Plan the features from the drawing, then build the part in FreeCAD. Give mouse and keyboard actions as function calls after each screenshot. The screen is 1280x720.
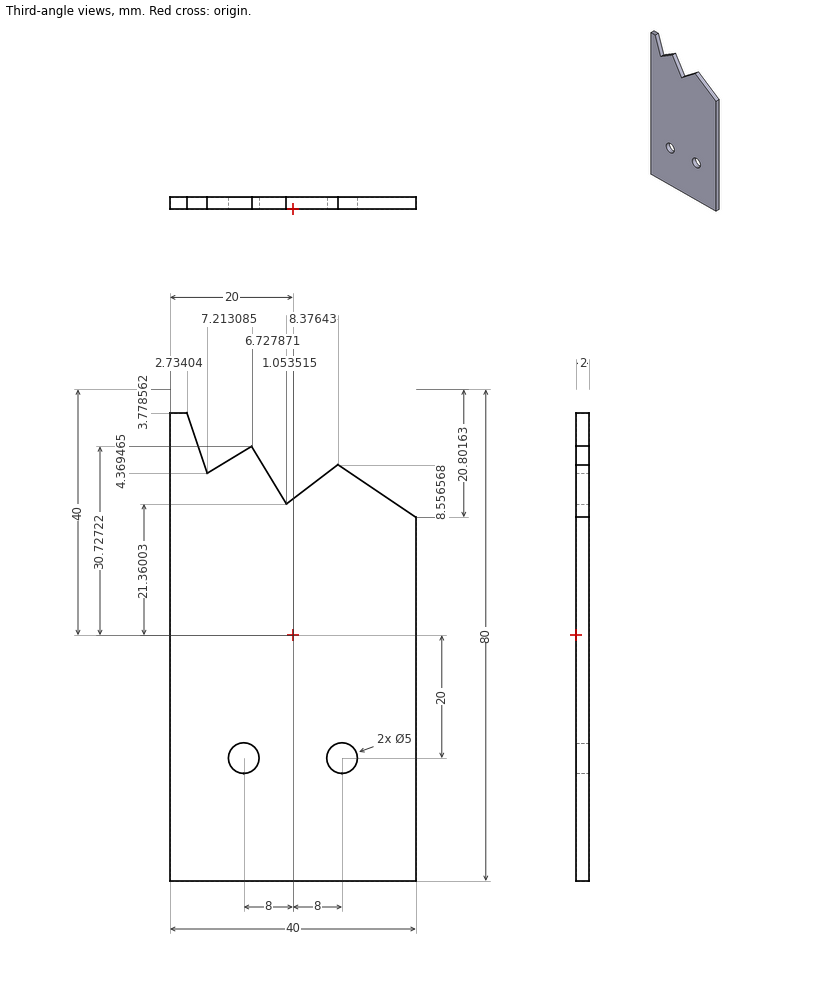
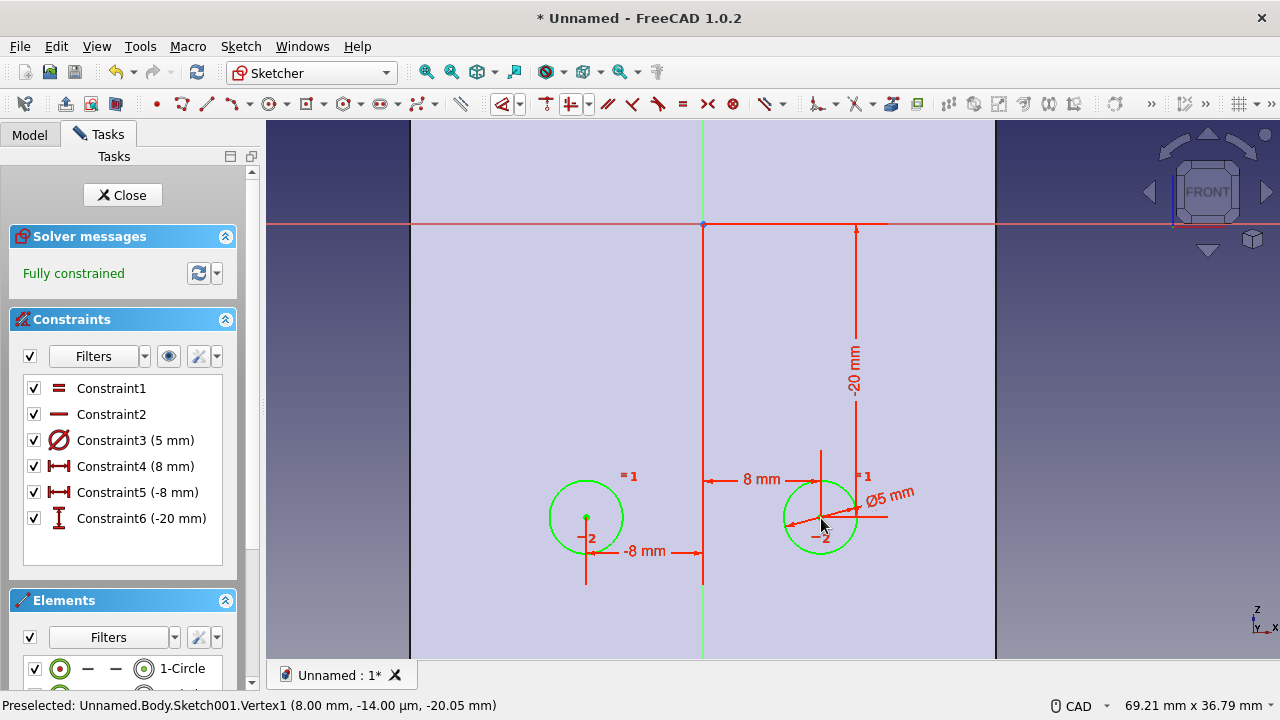
click(123, 195)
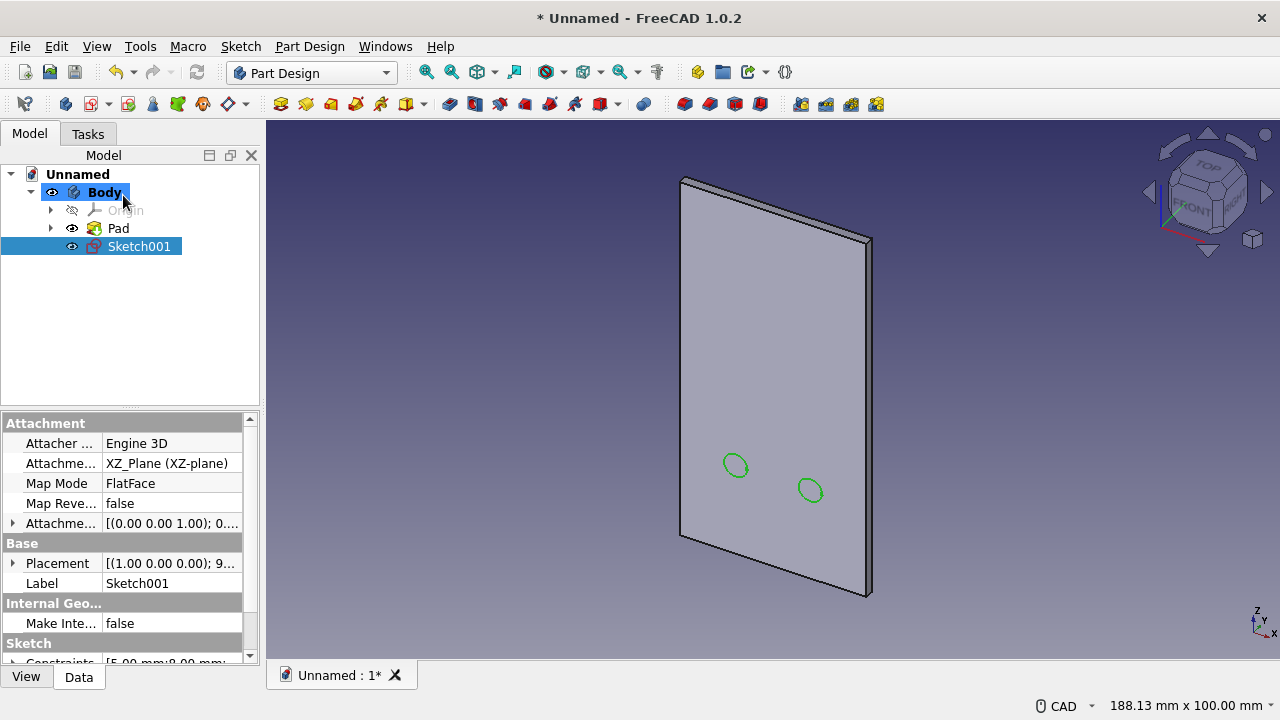
click(450, 104)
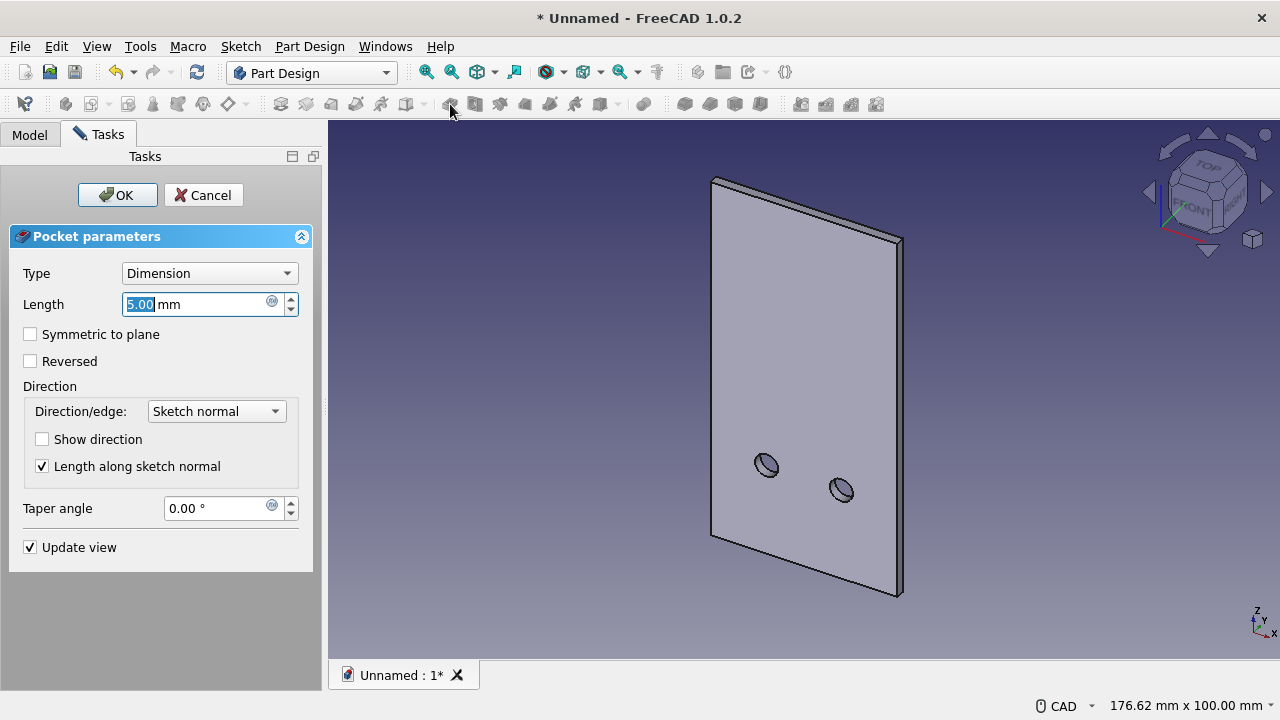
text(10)
key(Tab)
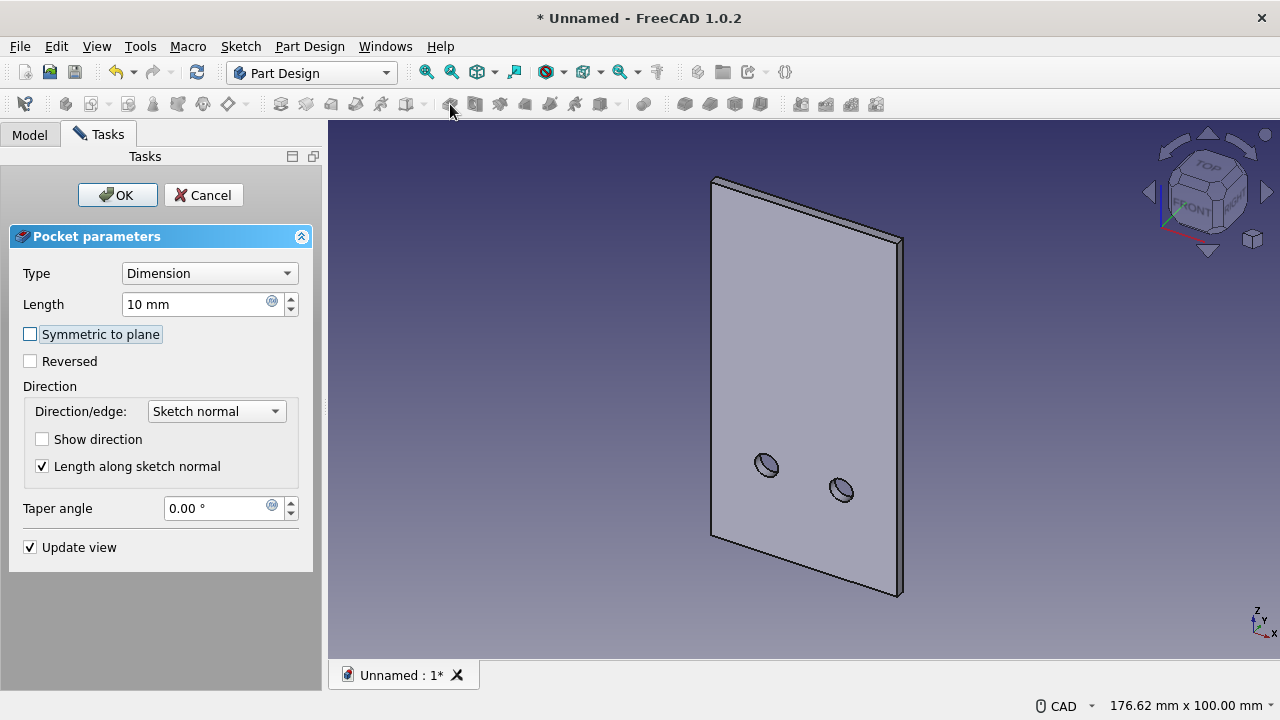
click(118, 195)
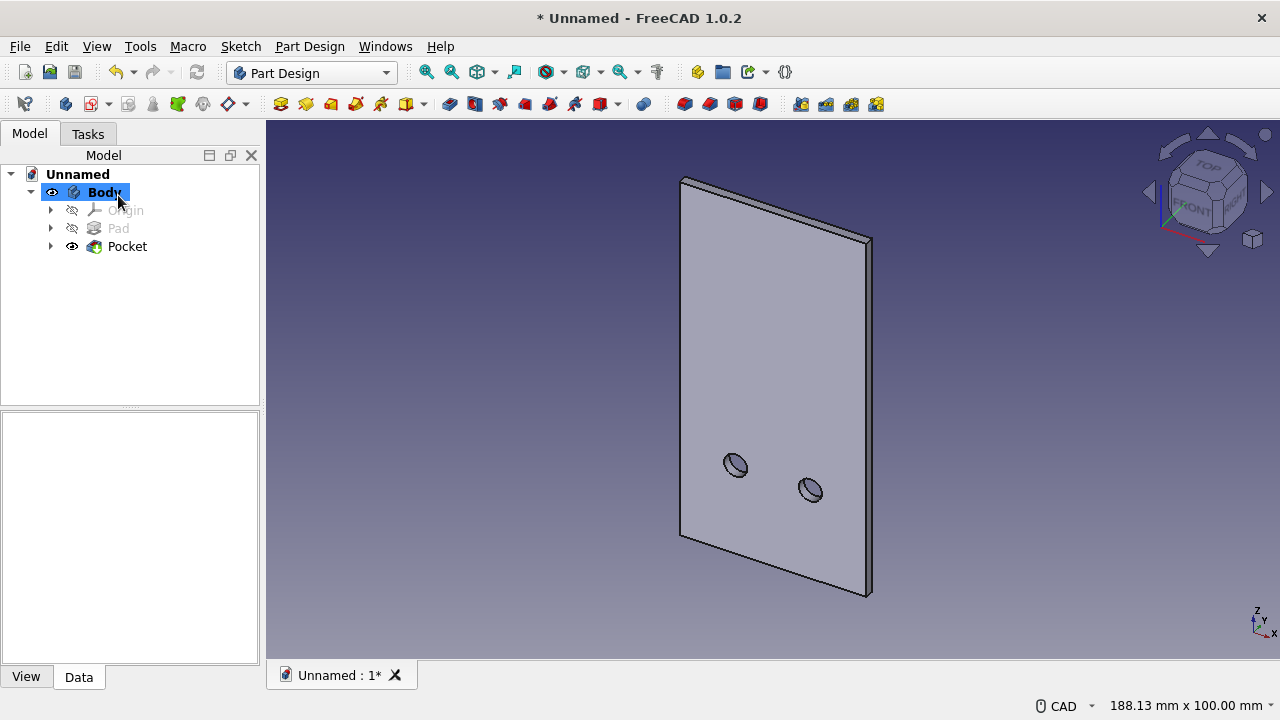
key(4)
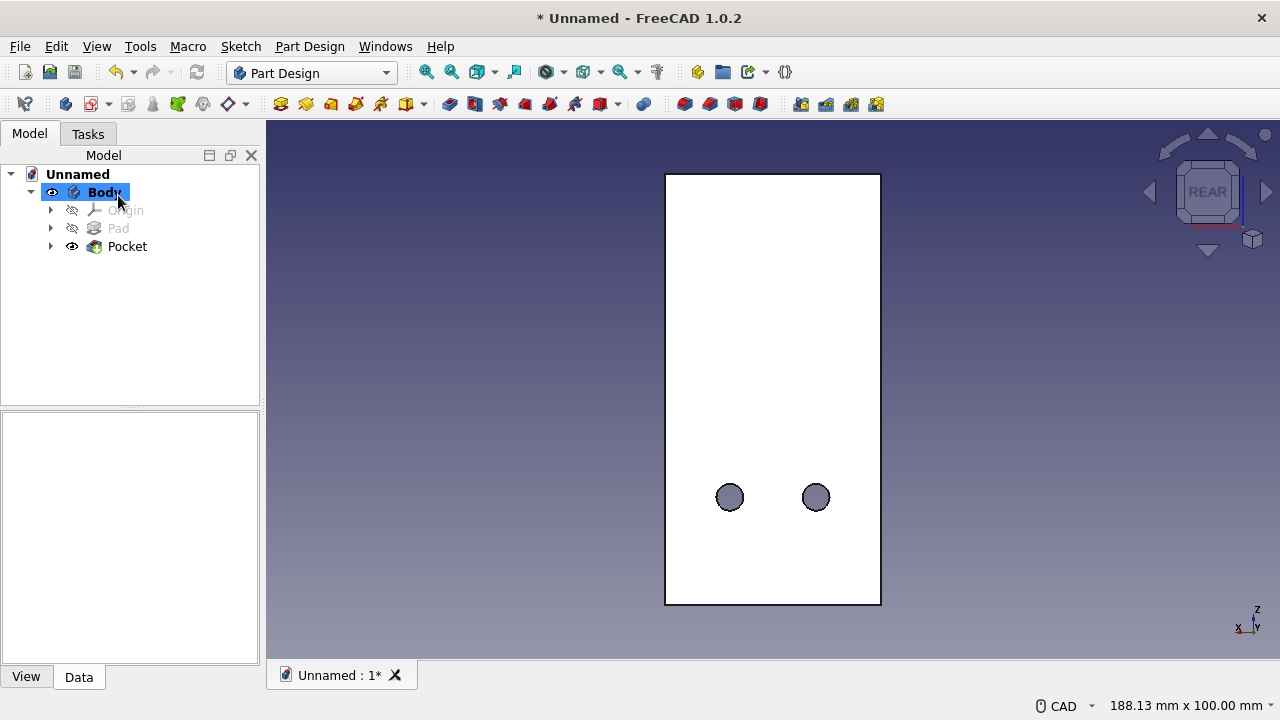
click(773, 327)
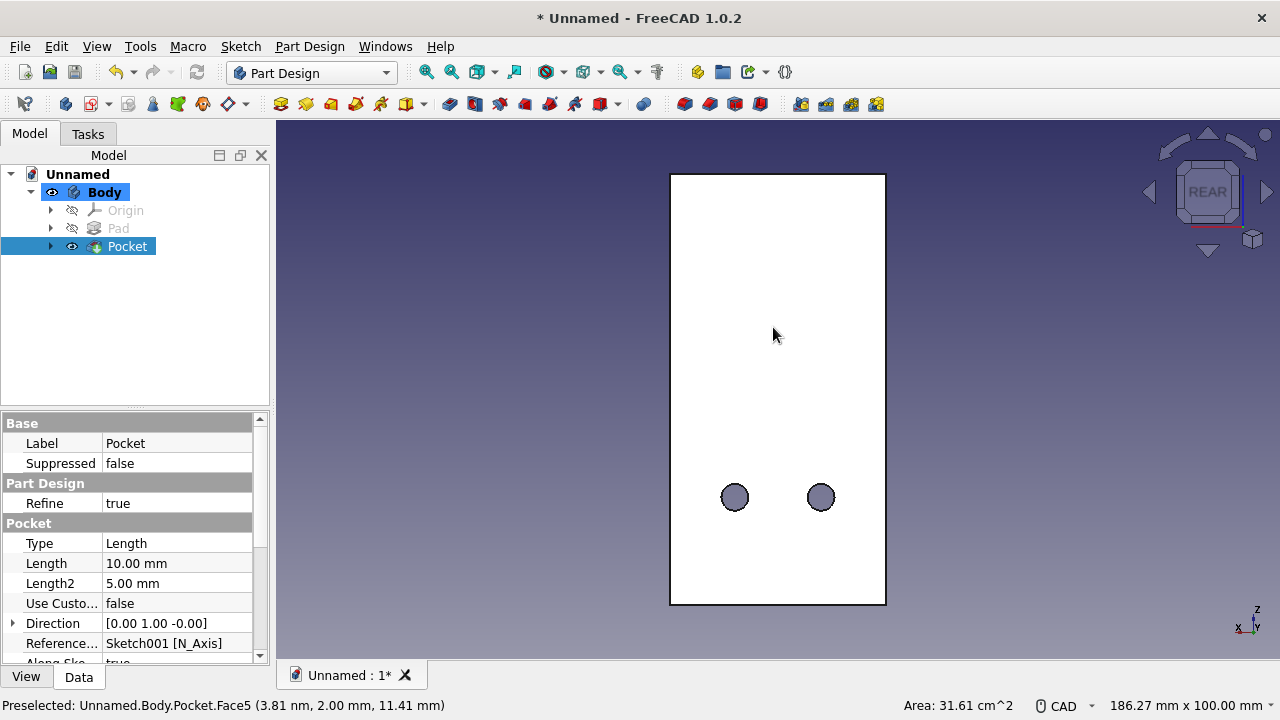
click(90, 104)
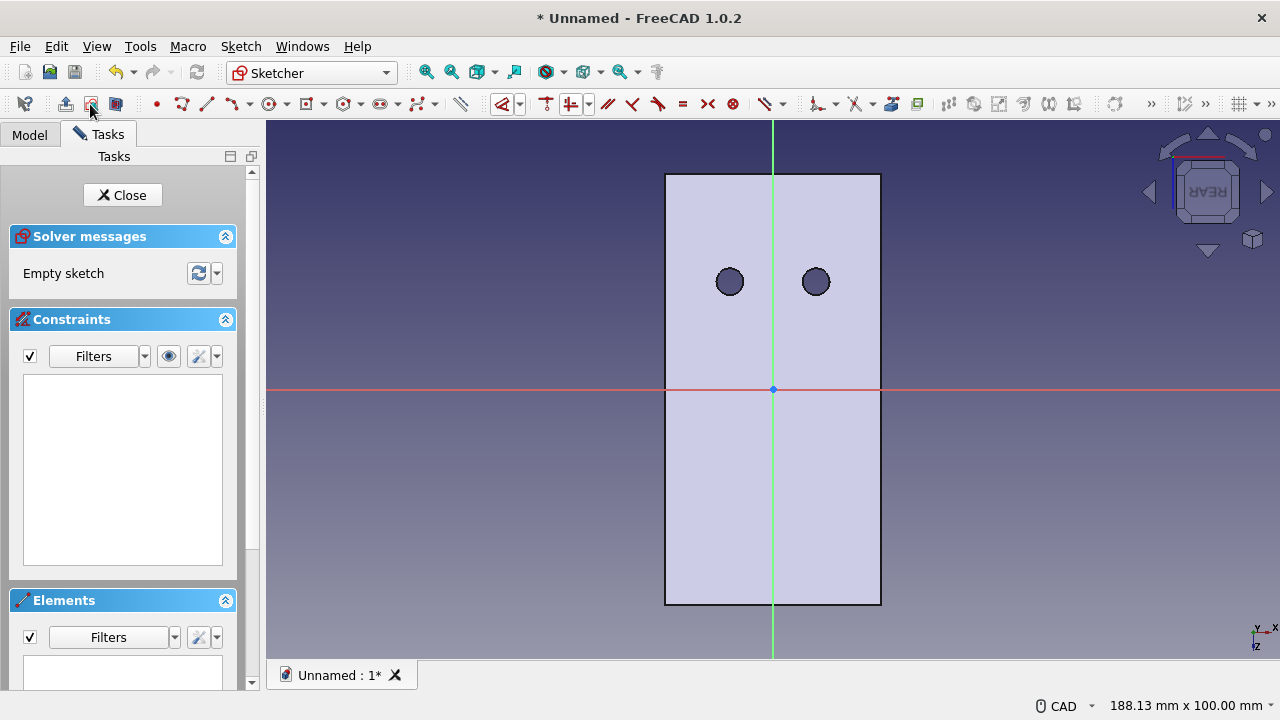
scroll(912, 631, up, 2)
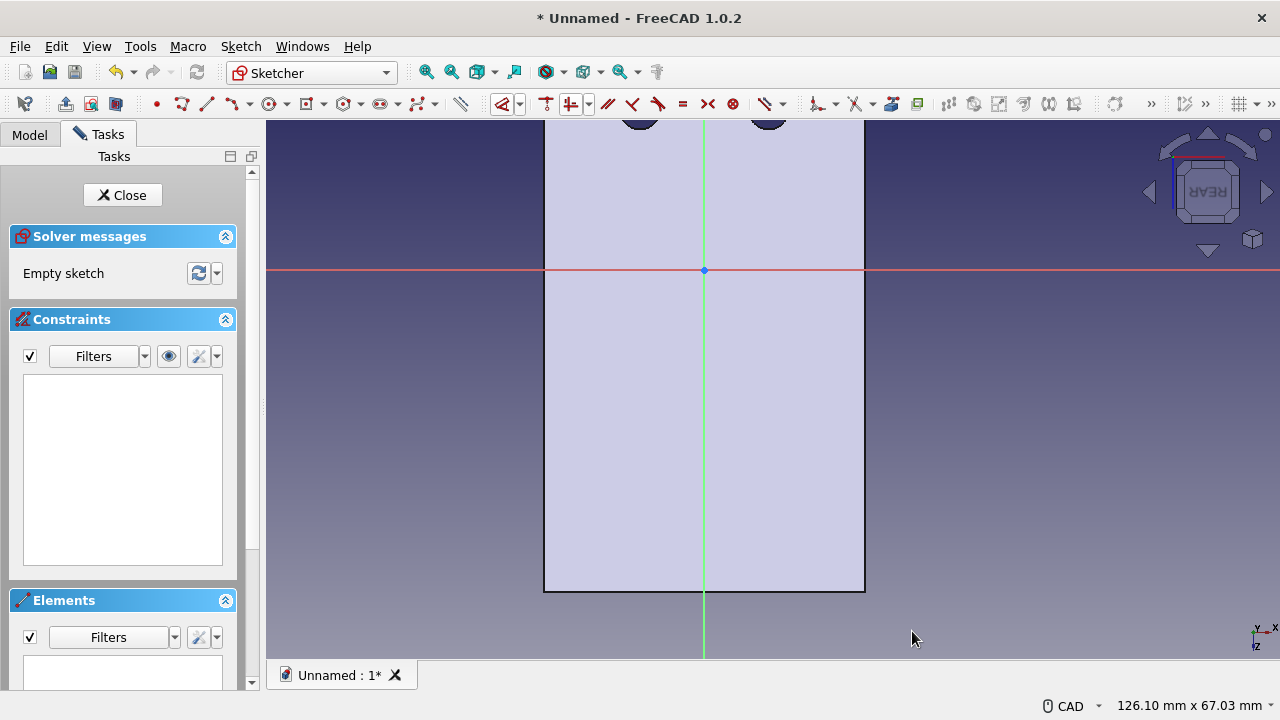
click(182, 104)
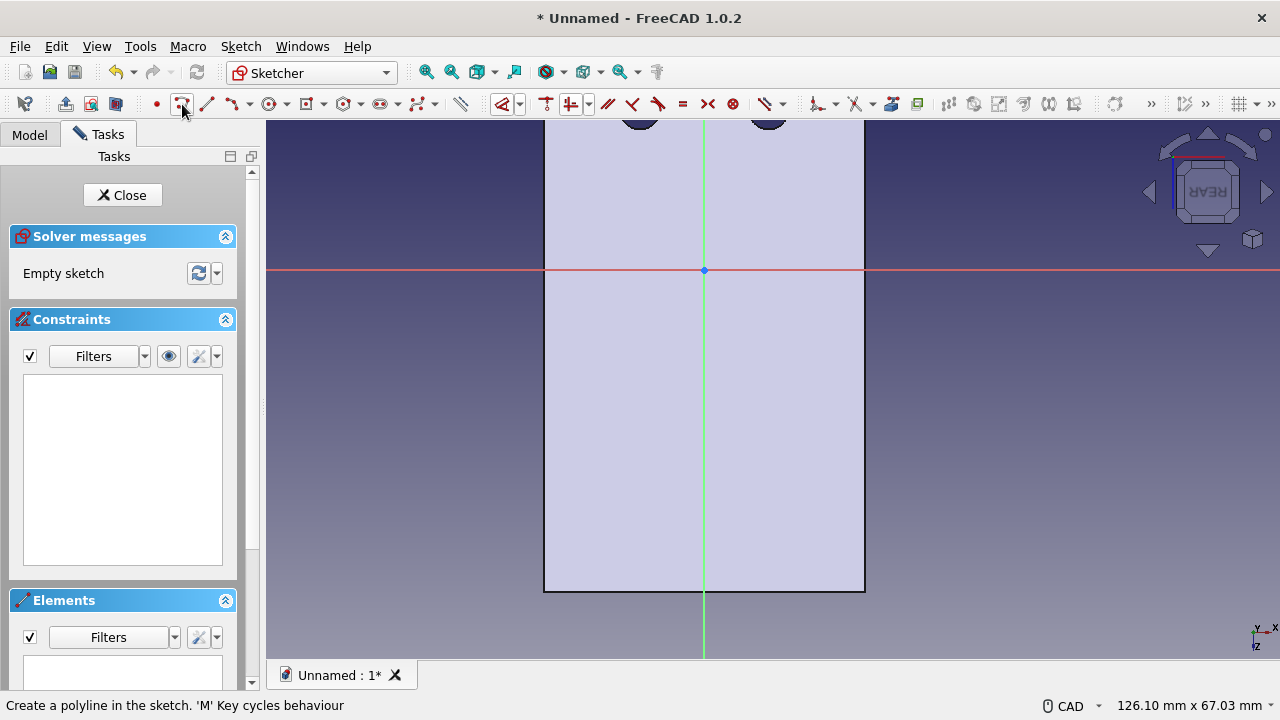
scroll(696, 442, up, 4)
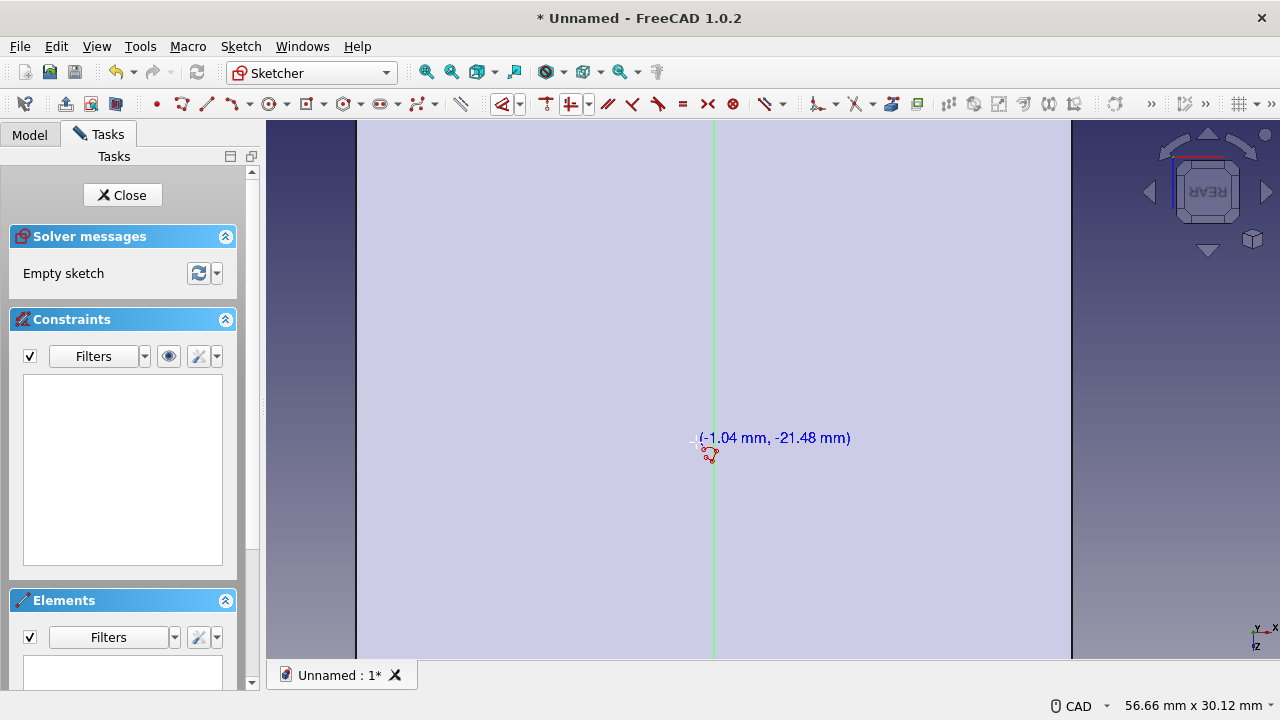
click(695, 441)
click(594, 609)
click(465, 531)